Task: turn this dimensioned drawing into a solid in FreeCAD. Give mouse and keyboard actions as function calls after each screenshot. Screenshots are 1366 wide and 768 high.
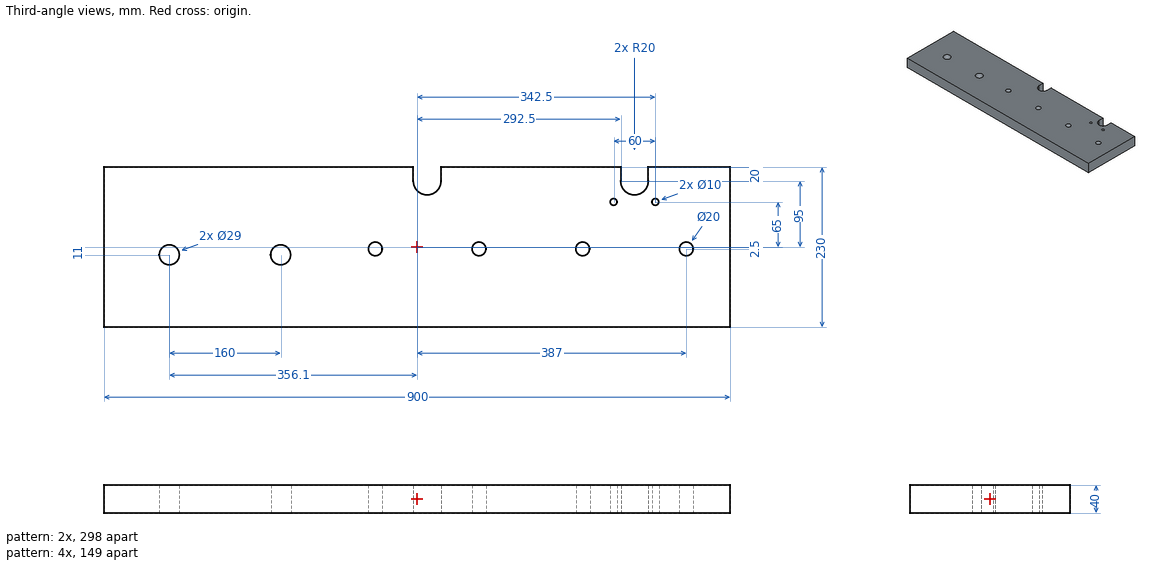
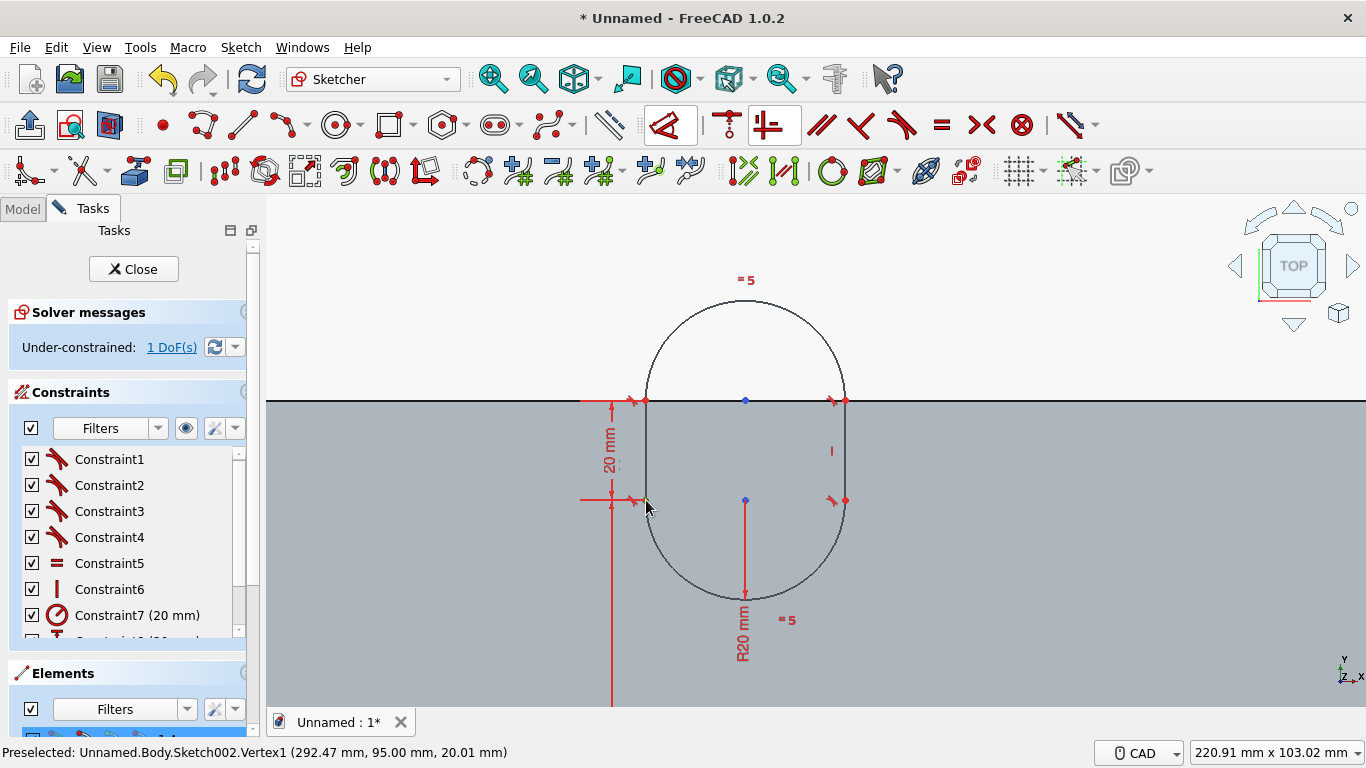
key(l)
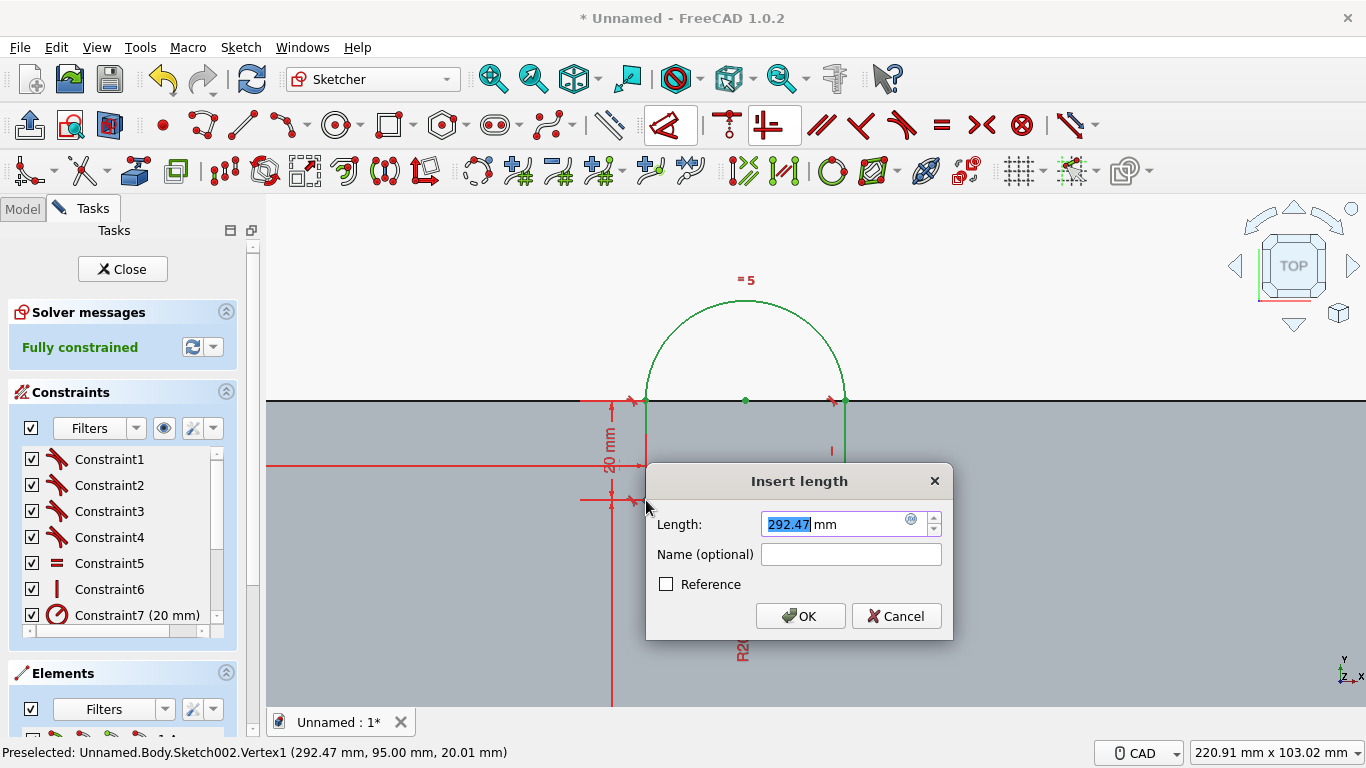
text(292.5)
key(Return)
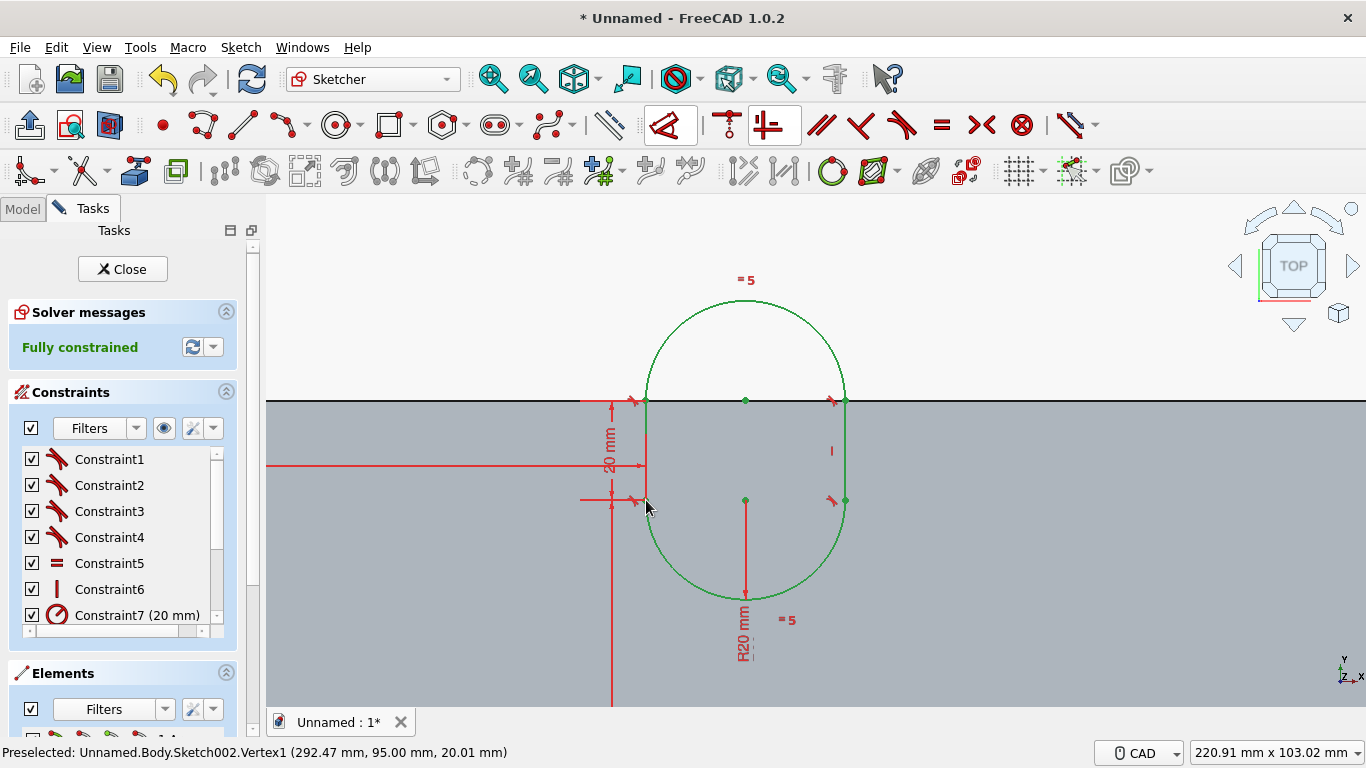
click(123, 269)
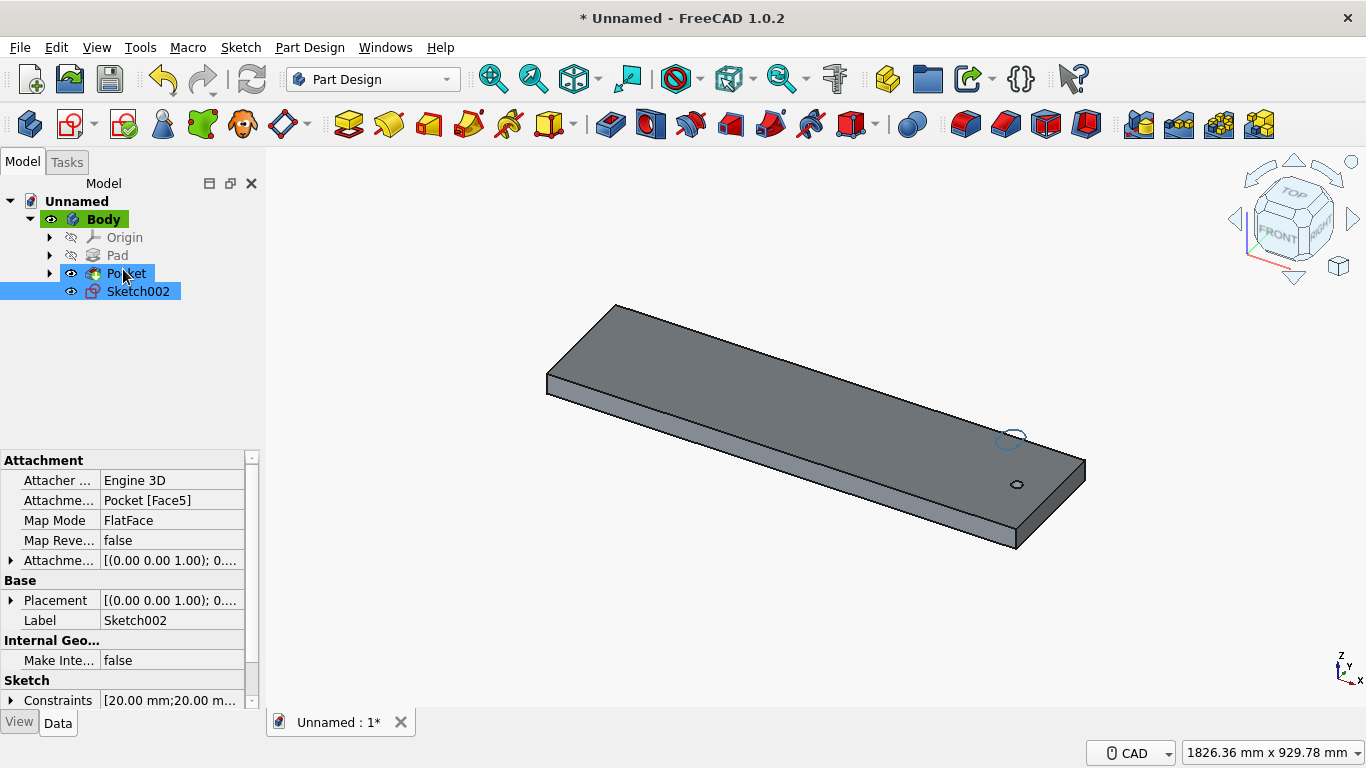
click(612, 124)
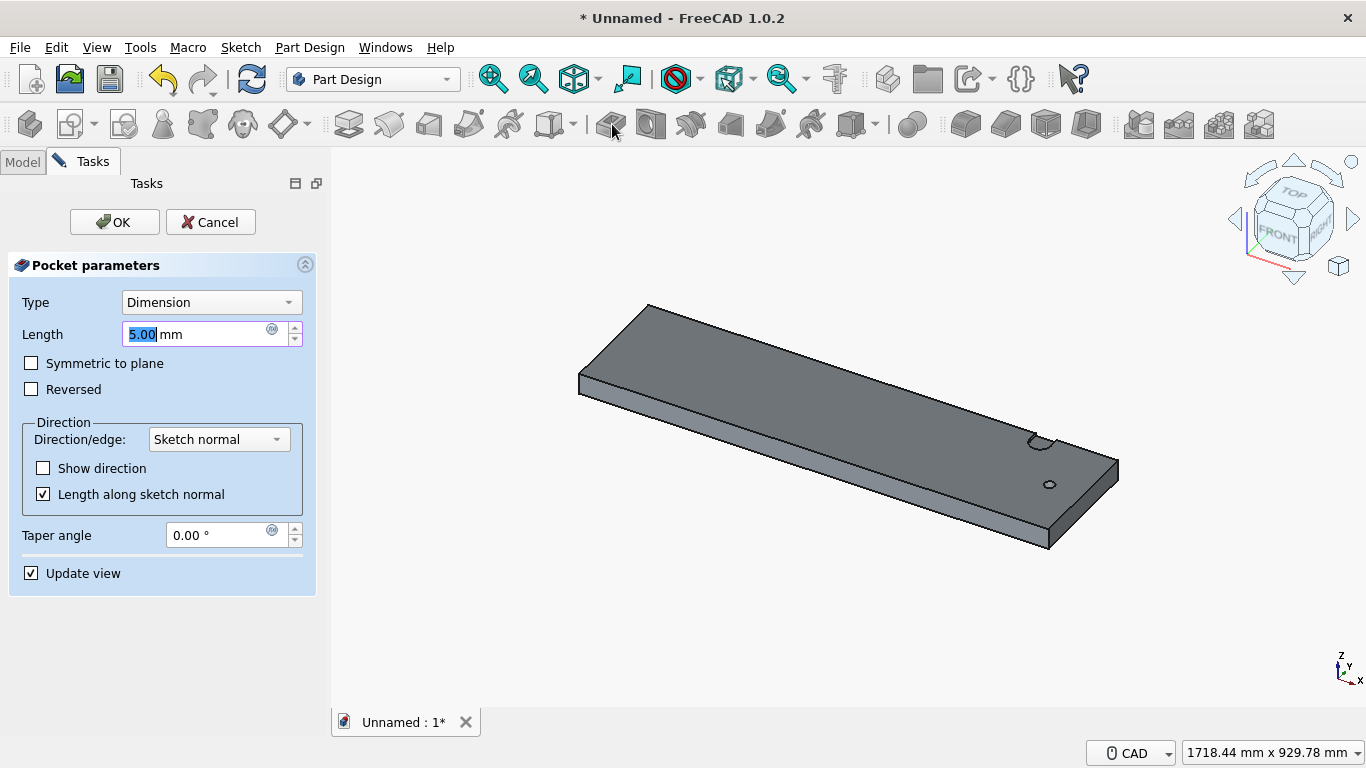
click(212, 302)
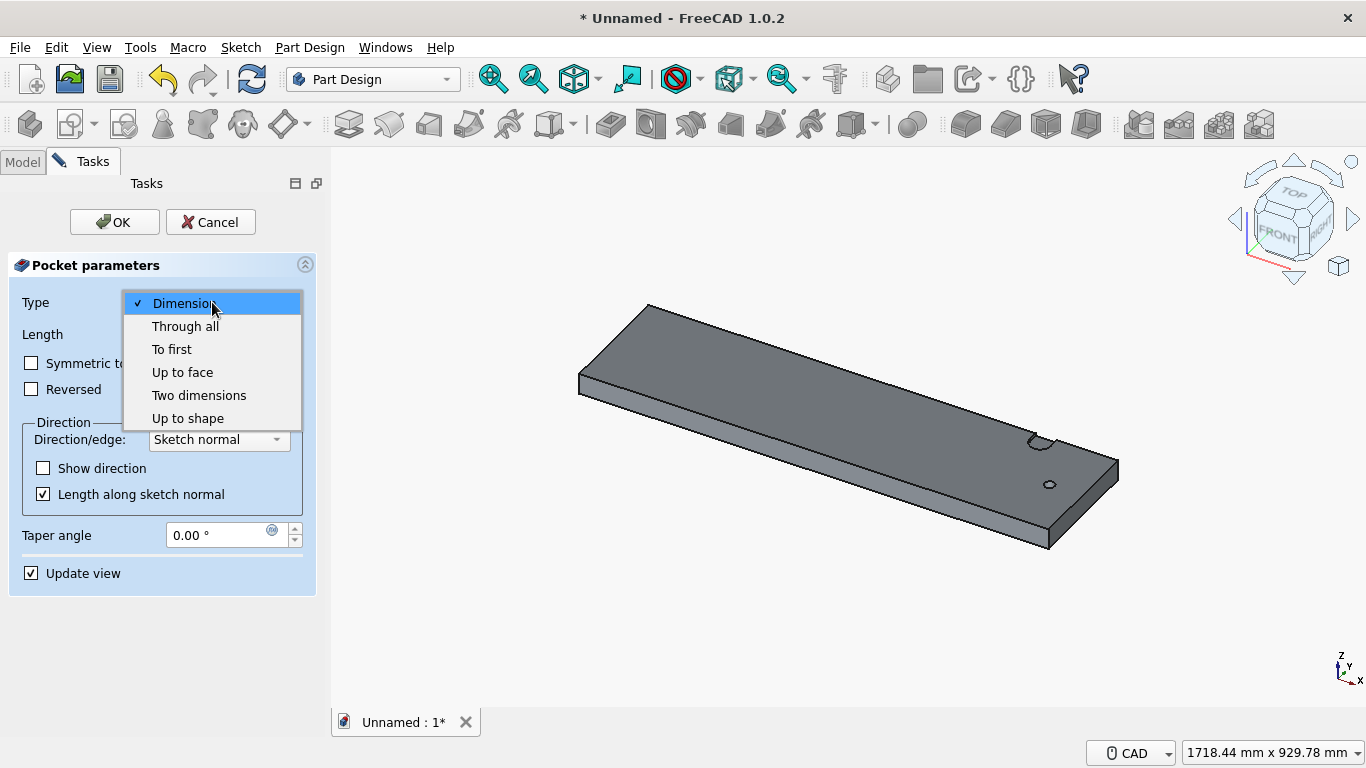
click(212, 326)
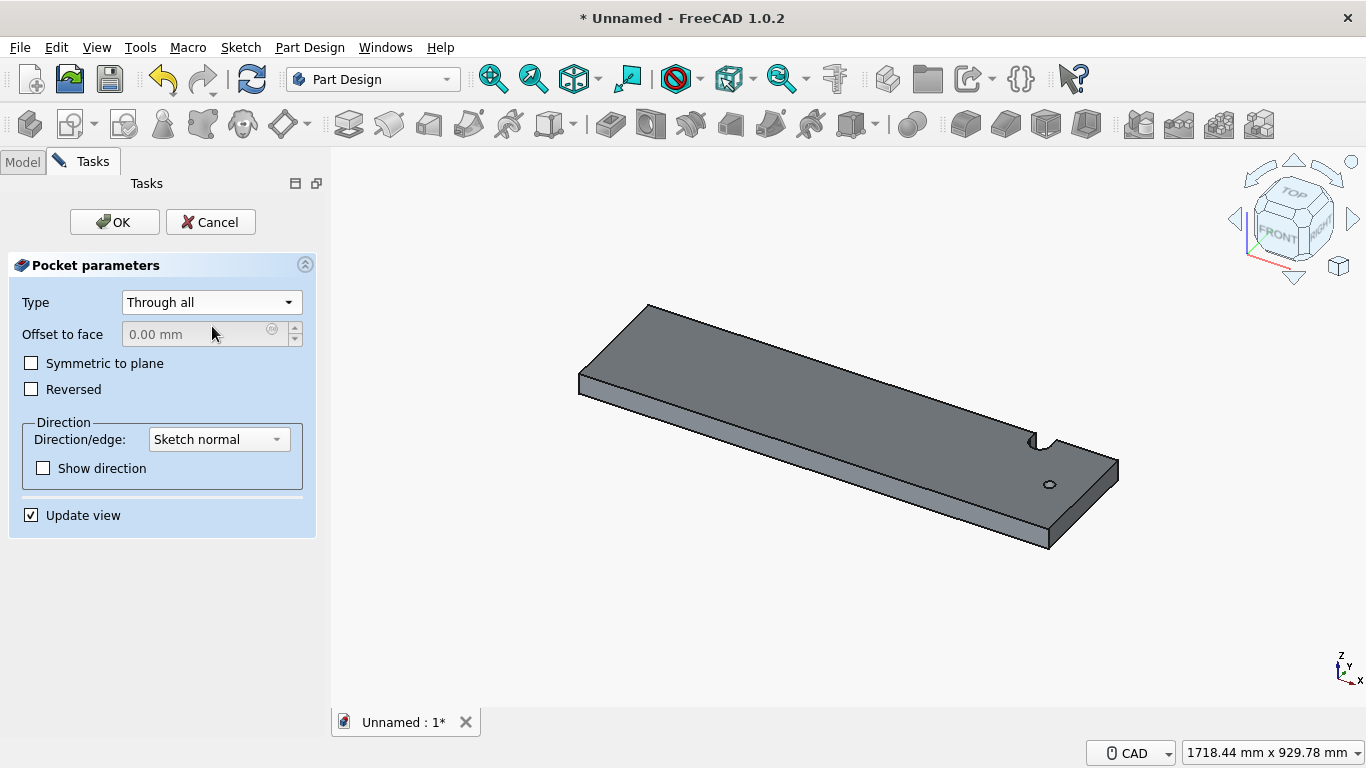
click(115, 222)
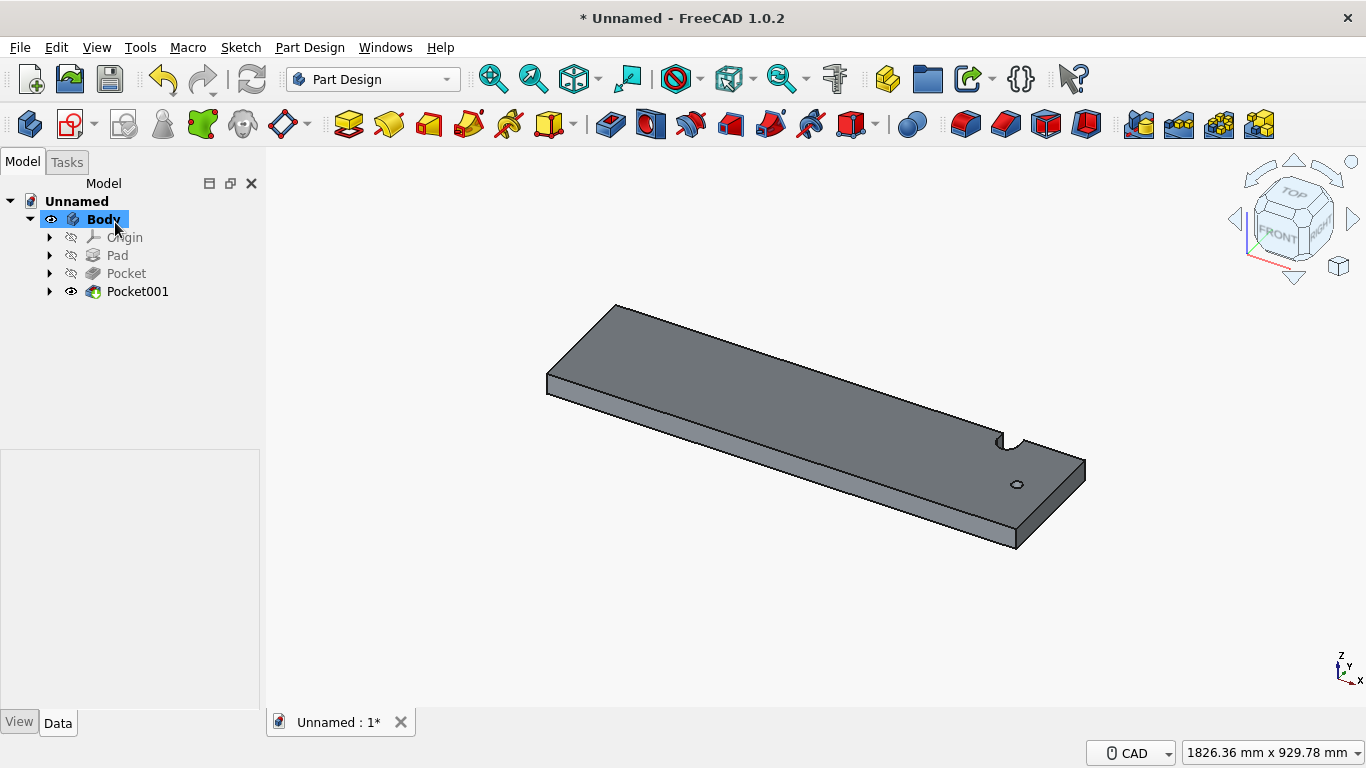
click(116, 291)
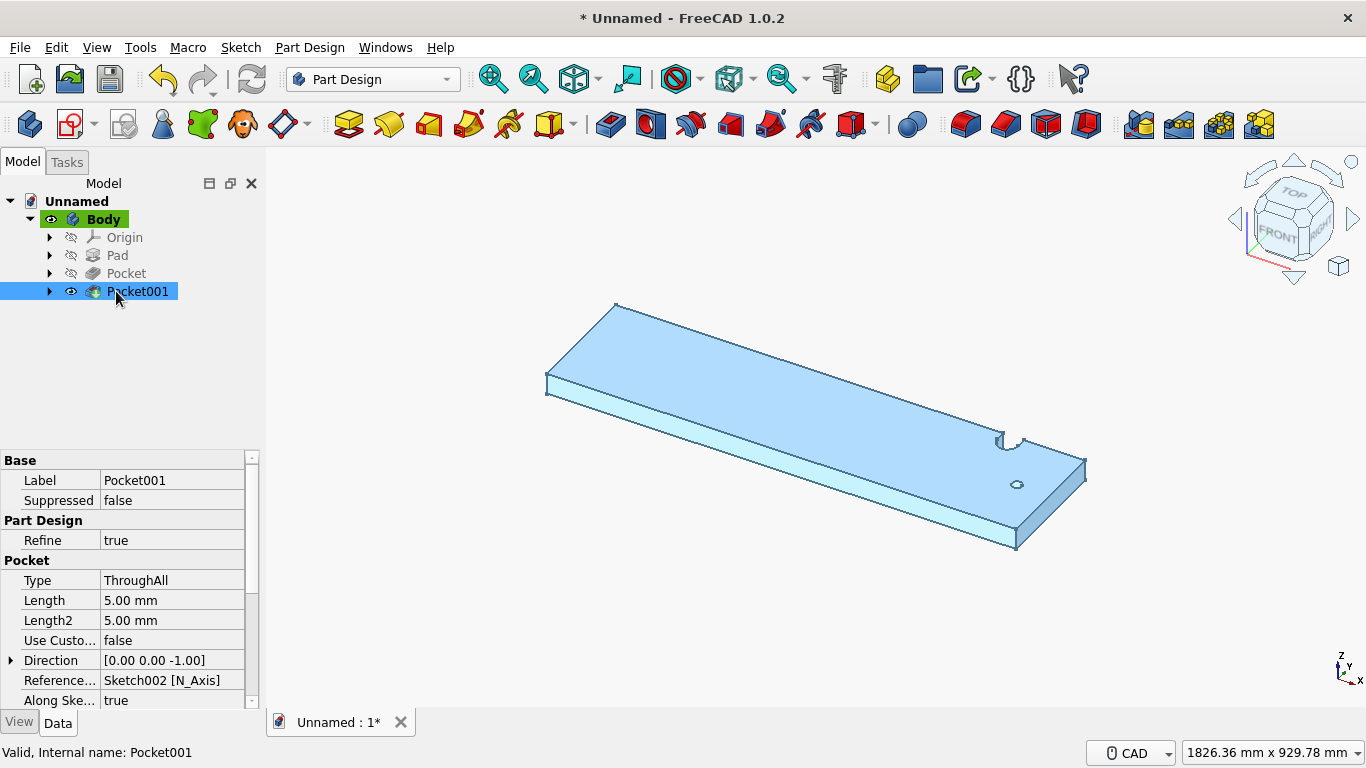
click(1180, 124)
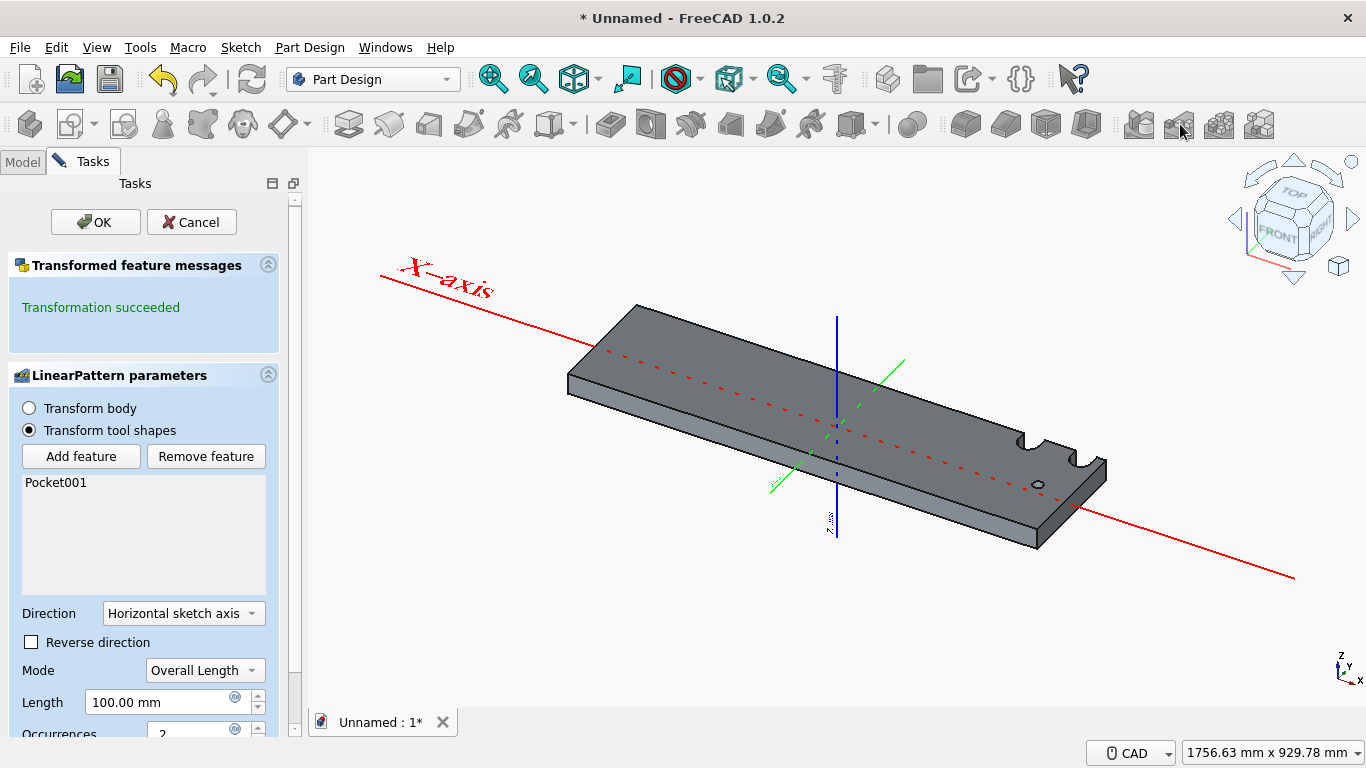
click(184, 614)